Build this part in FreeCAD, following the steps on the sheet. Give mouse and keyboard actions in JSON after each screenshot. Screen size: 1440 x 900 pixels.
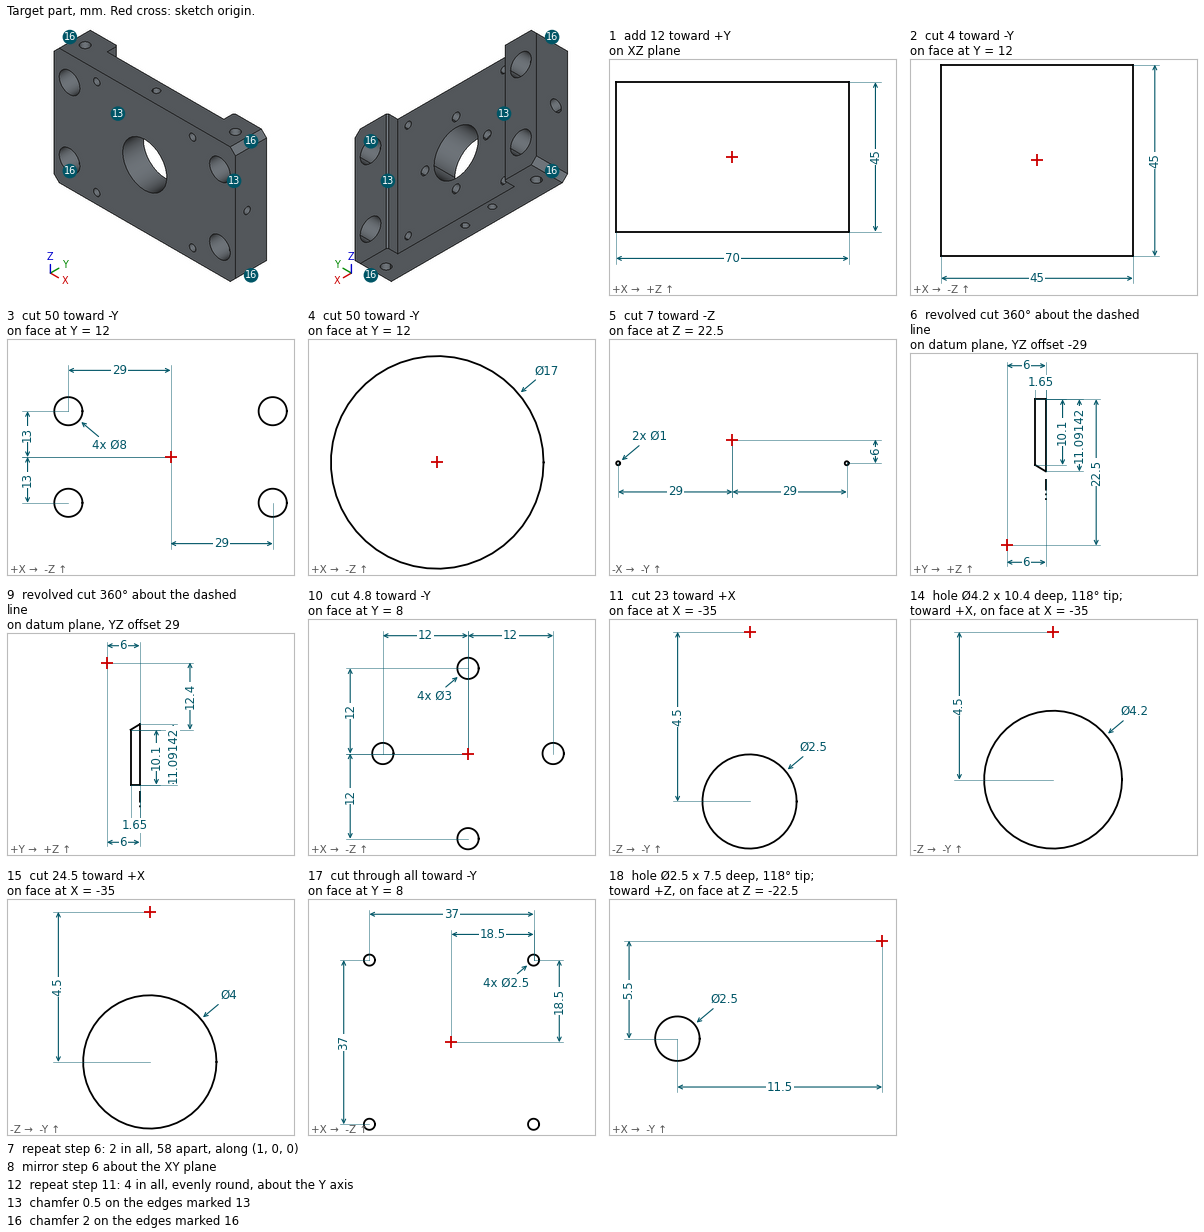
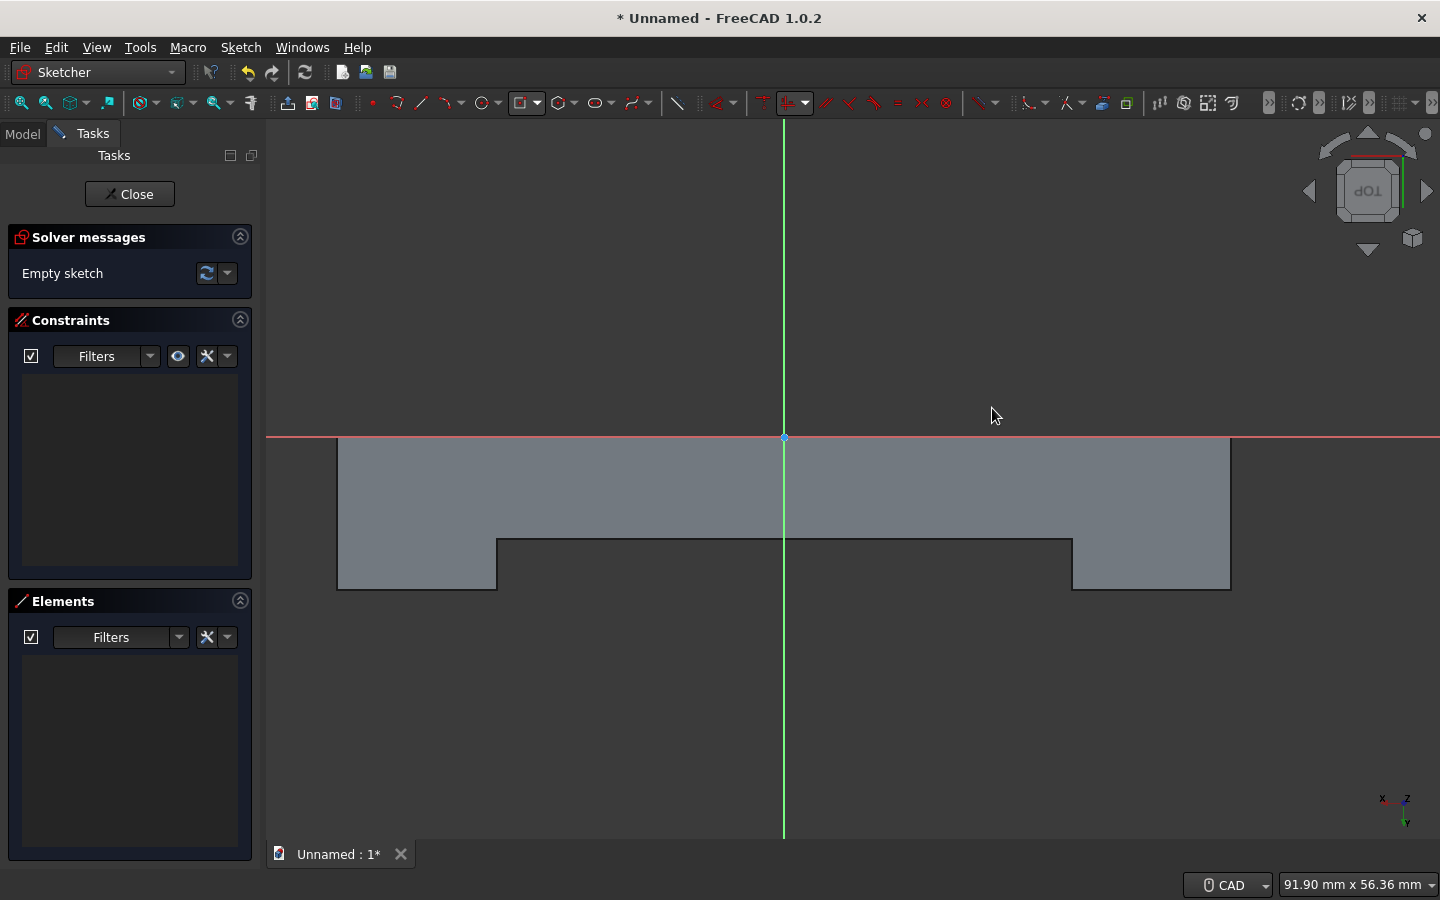
{"action": "left_click", "coordinate": [482, 104]}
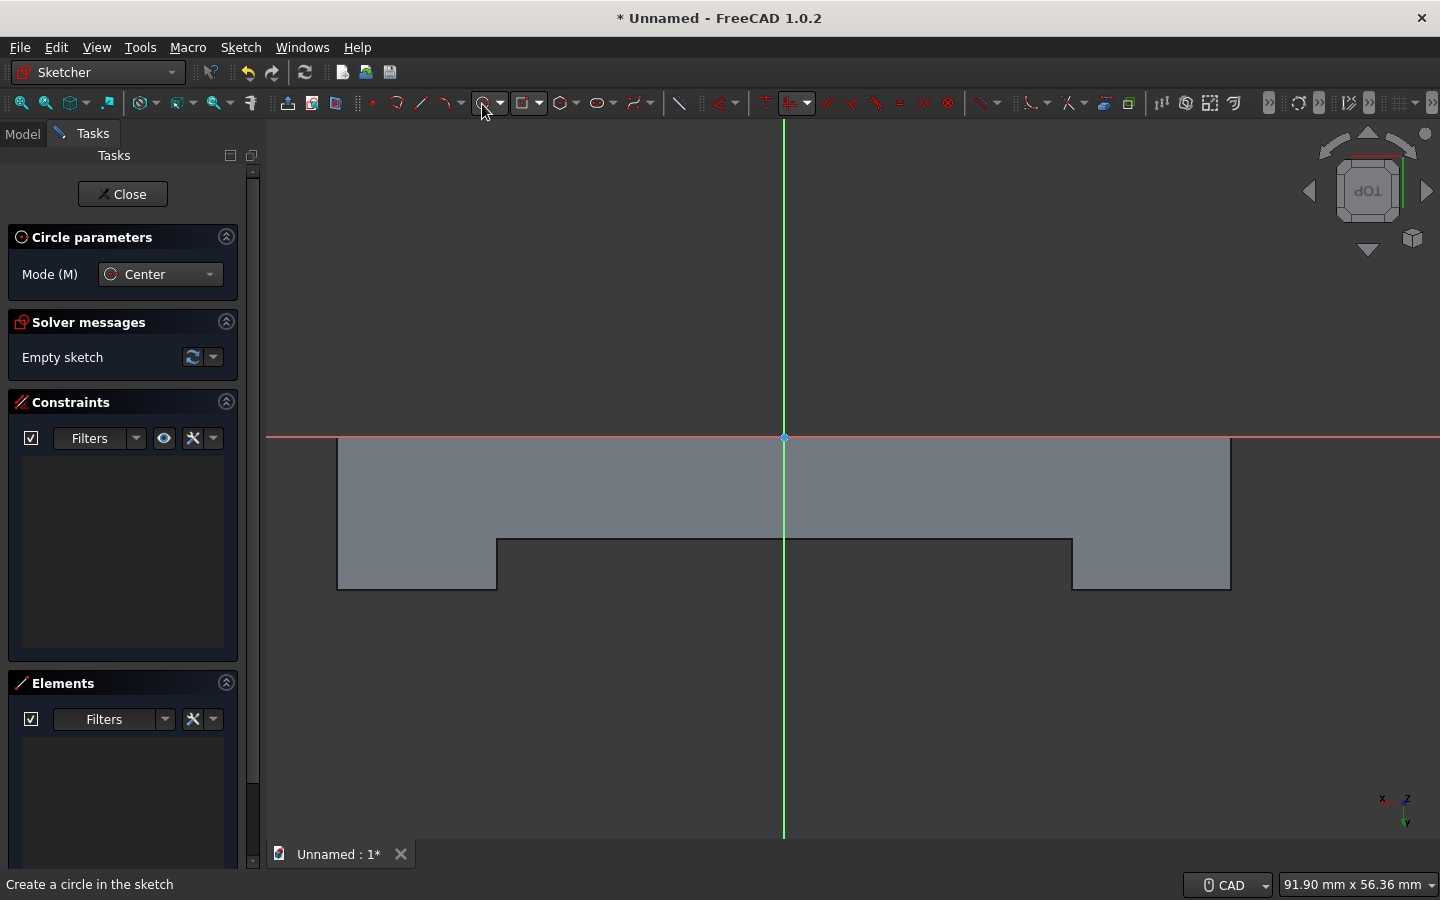
{"action": "scroll", "coordinate": [1155, 514], "scroll_direction": "up", "scroll_amount": 7}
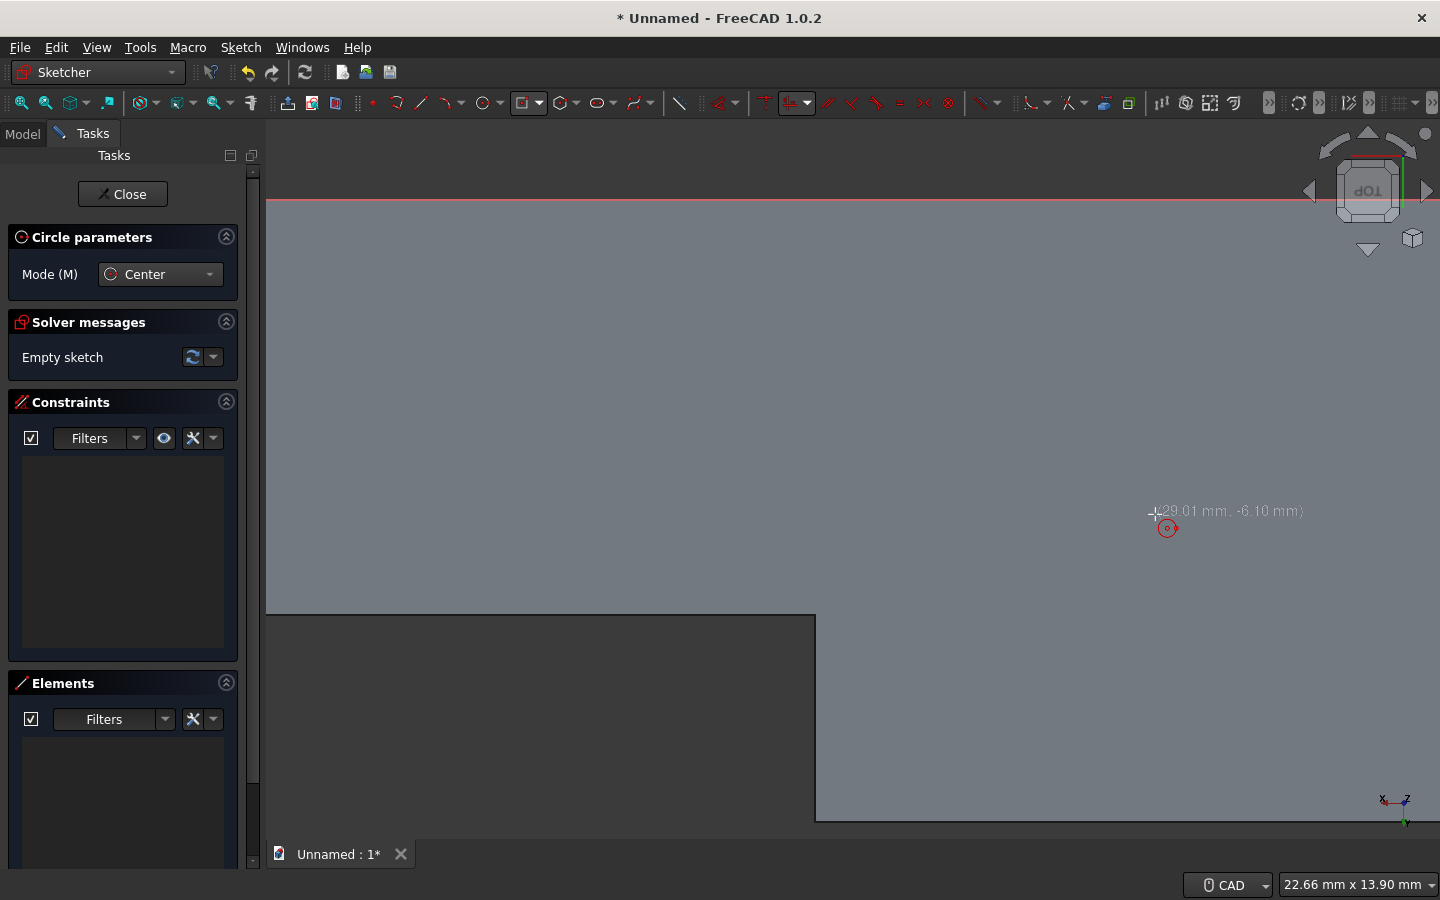
{"action": "scroll", "coordinate": [1156, 515], "scroll_direction": "down", "scroll_amount": 7}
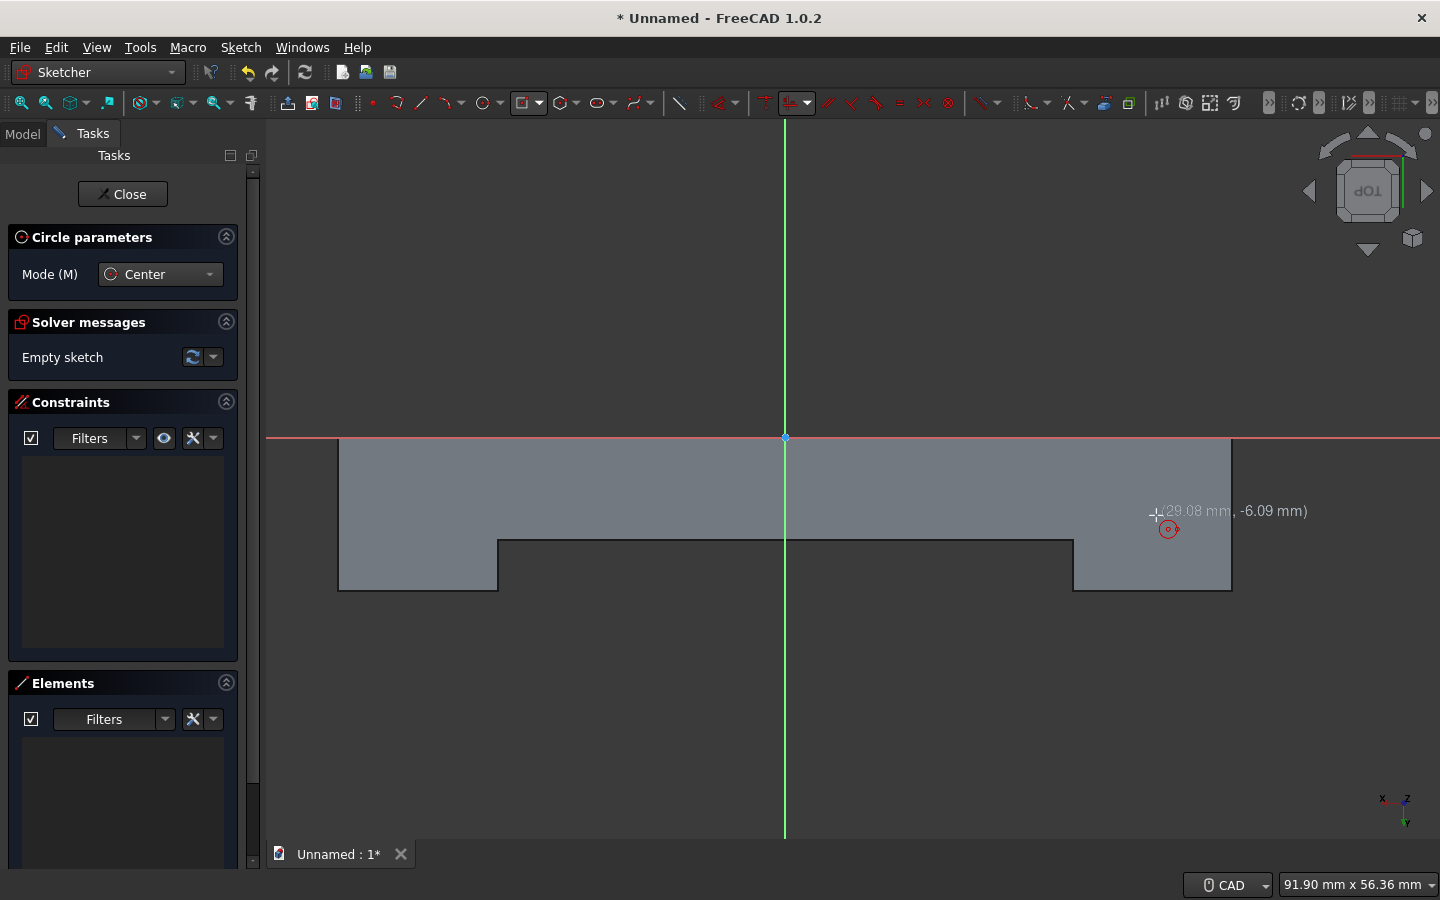
{"action": "left_click", "coordinate": [1156, 514]}
{"action": "mouse_move", "coordinate": [1160, 510]}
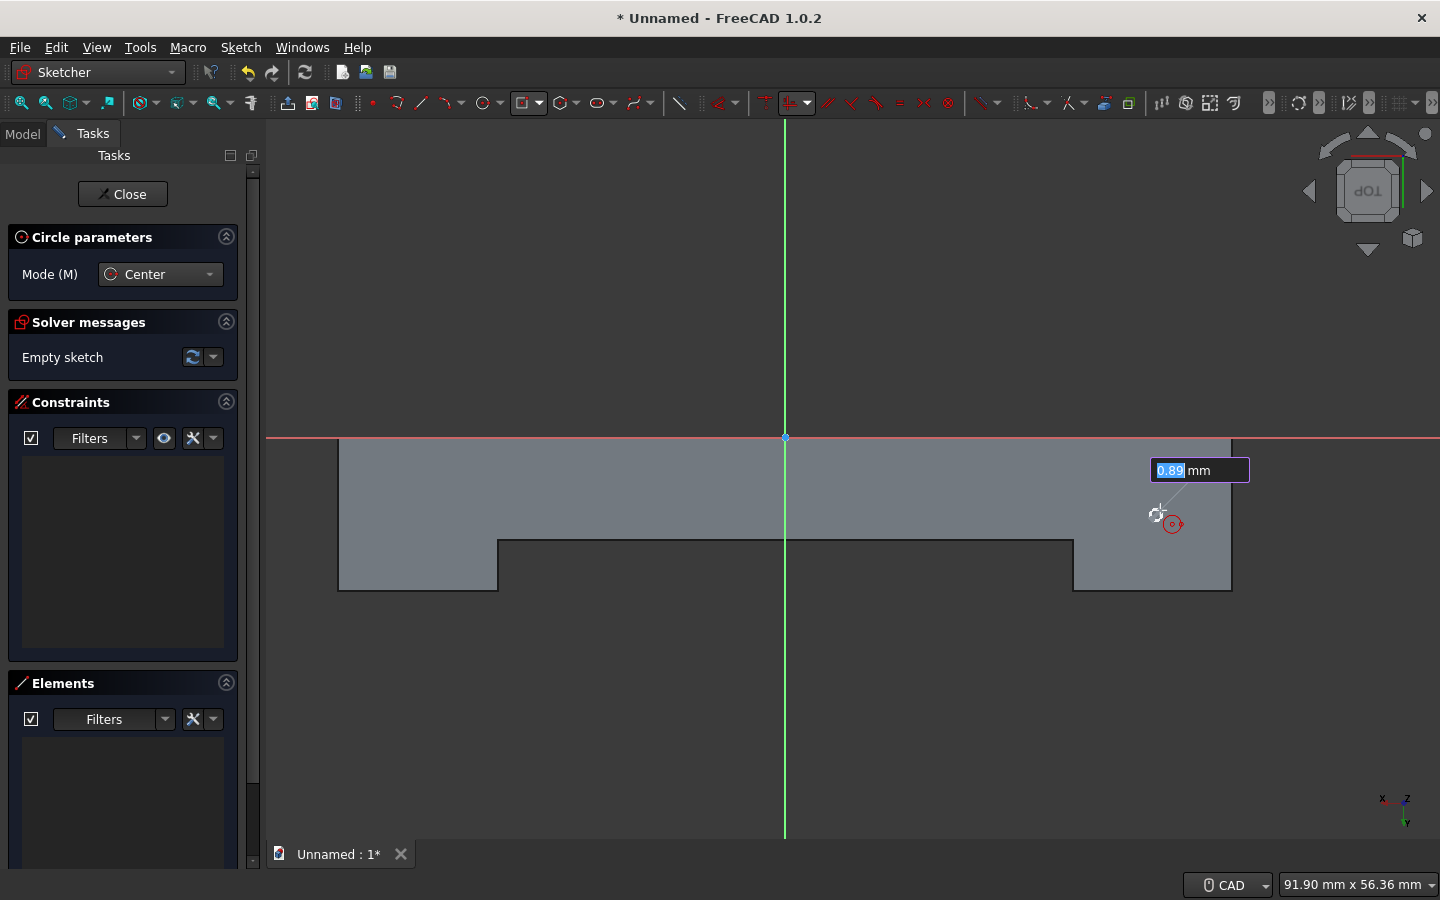
{"action": "type", "text": "1"}
{"action": "key", "text": "Return"}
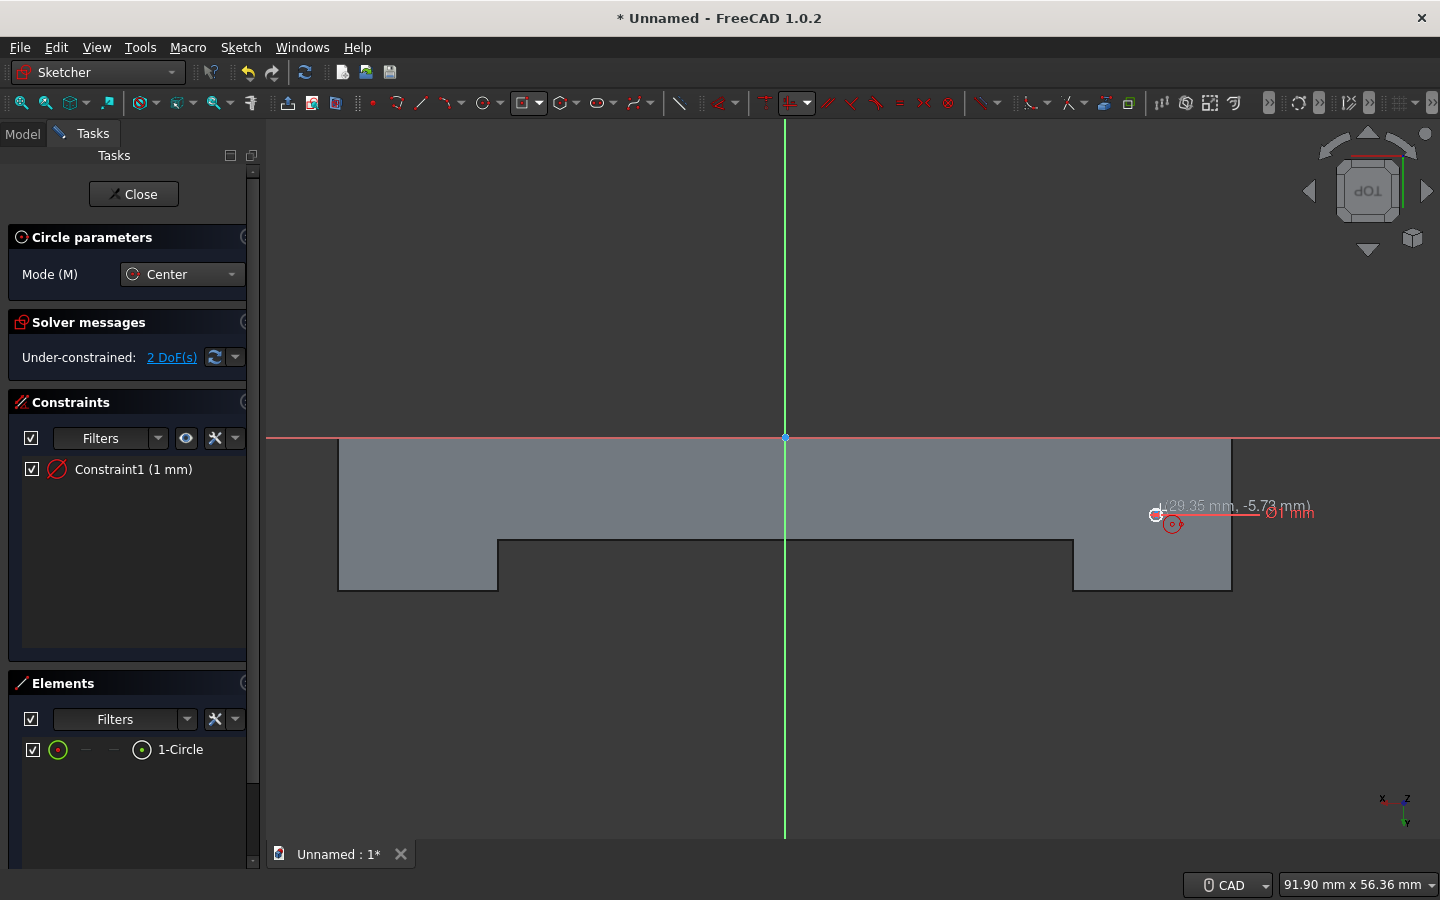
{"action": "scroll", "coordinate": [415, 514], "scroll_direction": "up", "scroll_amount": 7}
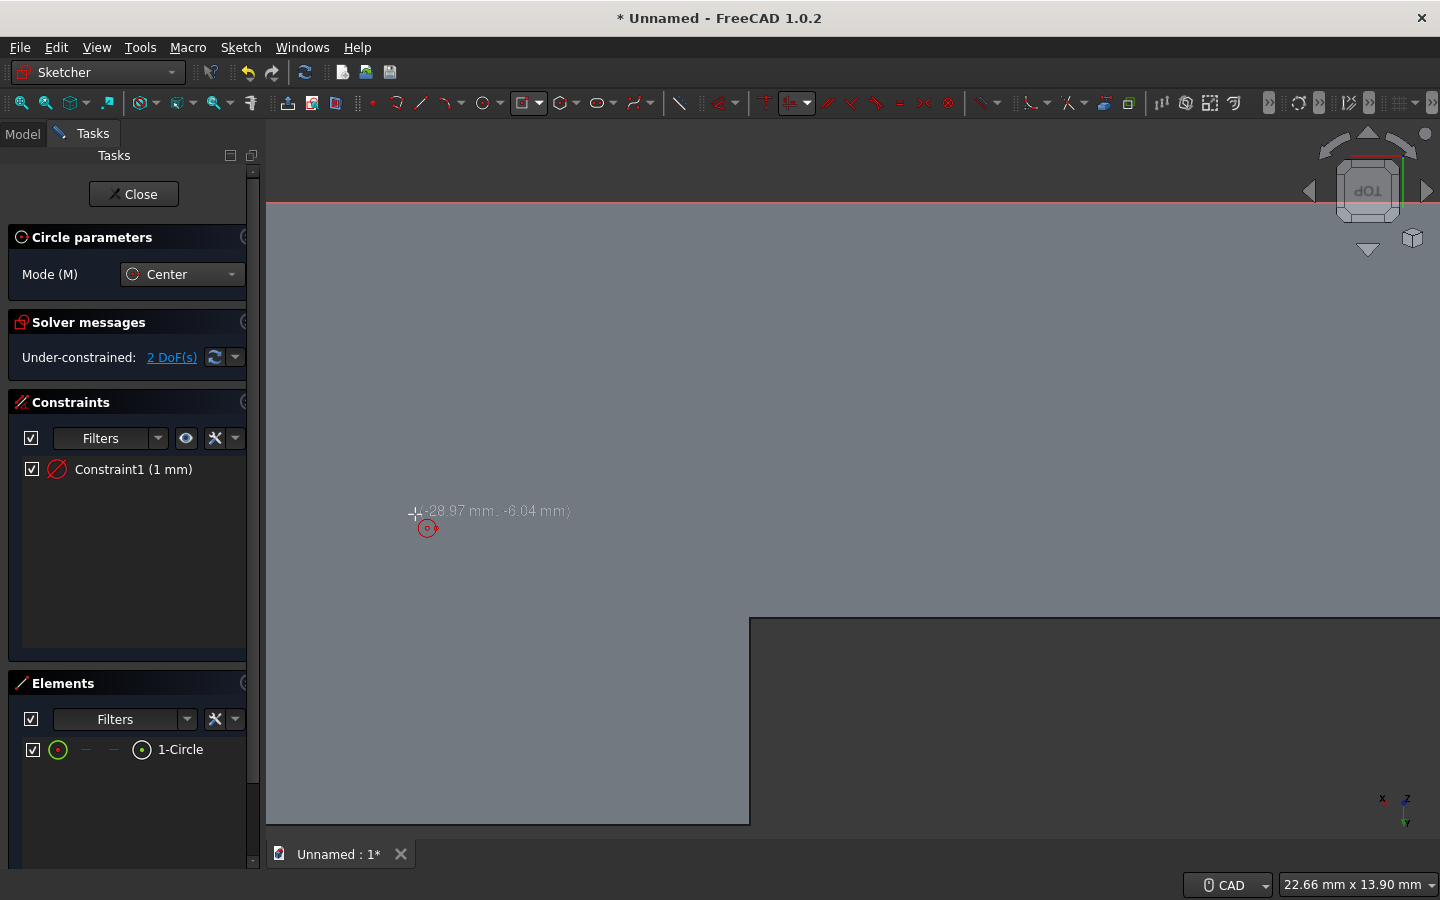
{"action": "scroll", "coordinate": [414, 514], "scroll_direction": "down", "scroll_amount": 7}